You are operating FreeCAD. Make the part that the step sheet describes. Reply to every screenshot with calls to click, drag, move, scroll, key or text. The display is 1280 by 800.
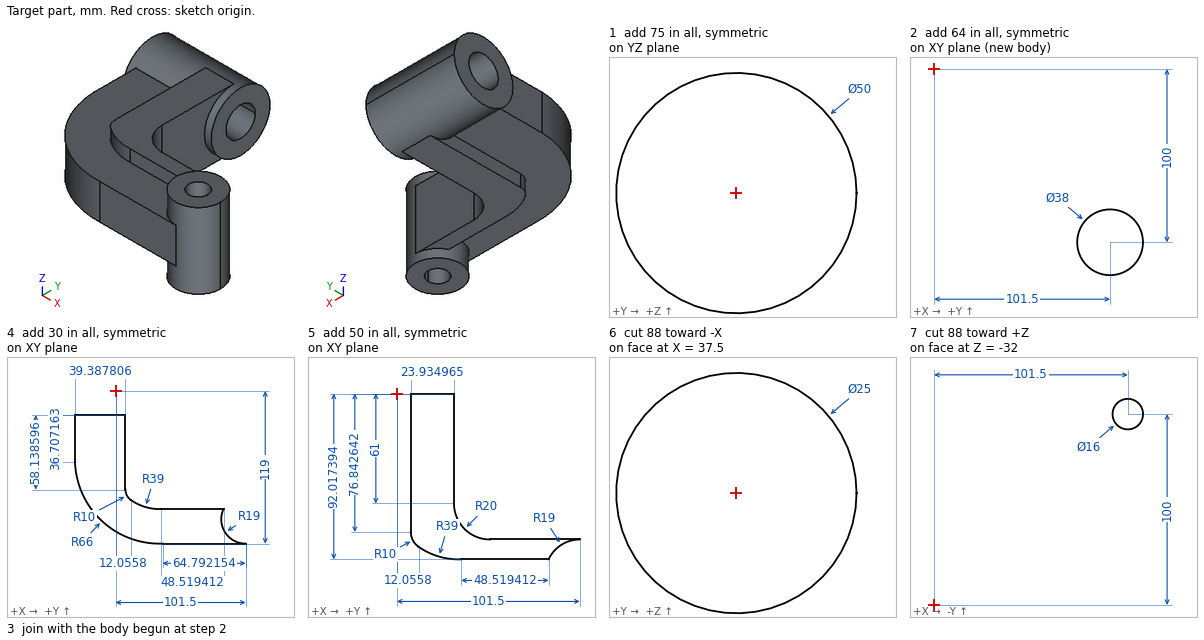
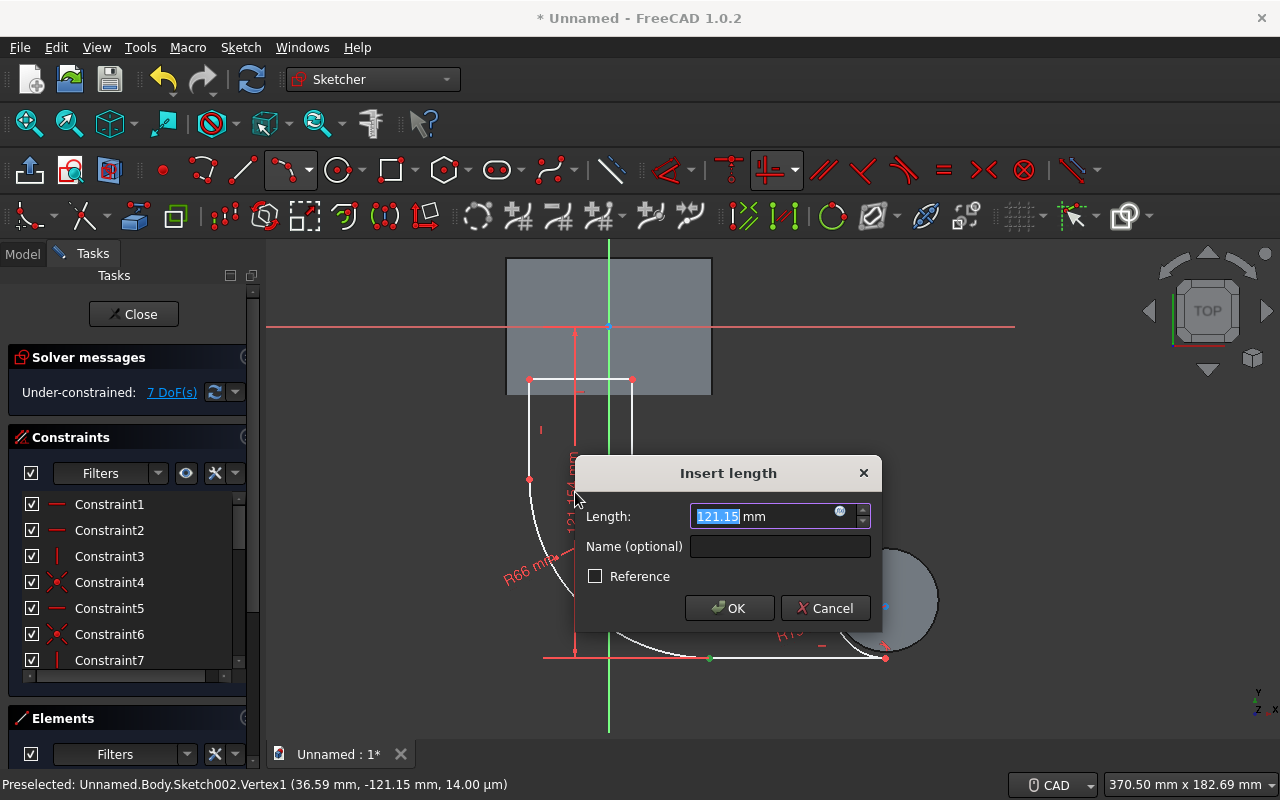
text(119)
key(Return)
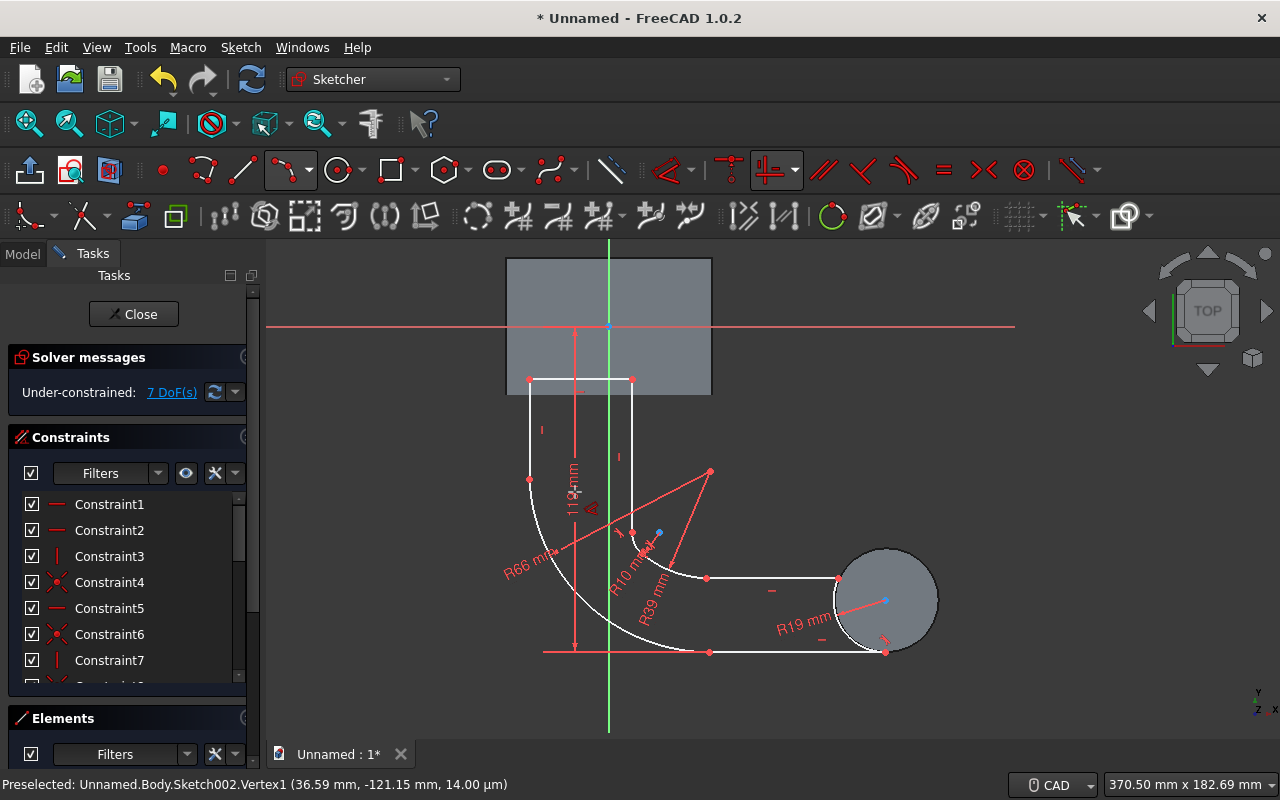
click(886, 652)
click(747, 686)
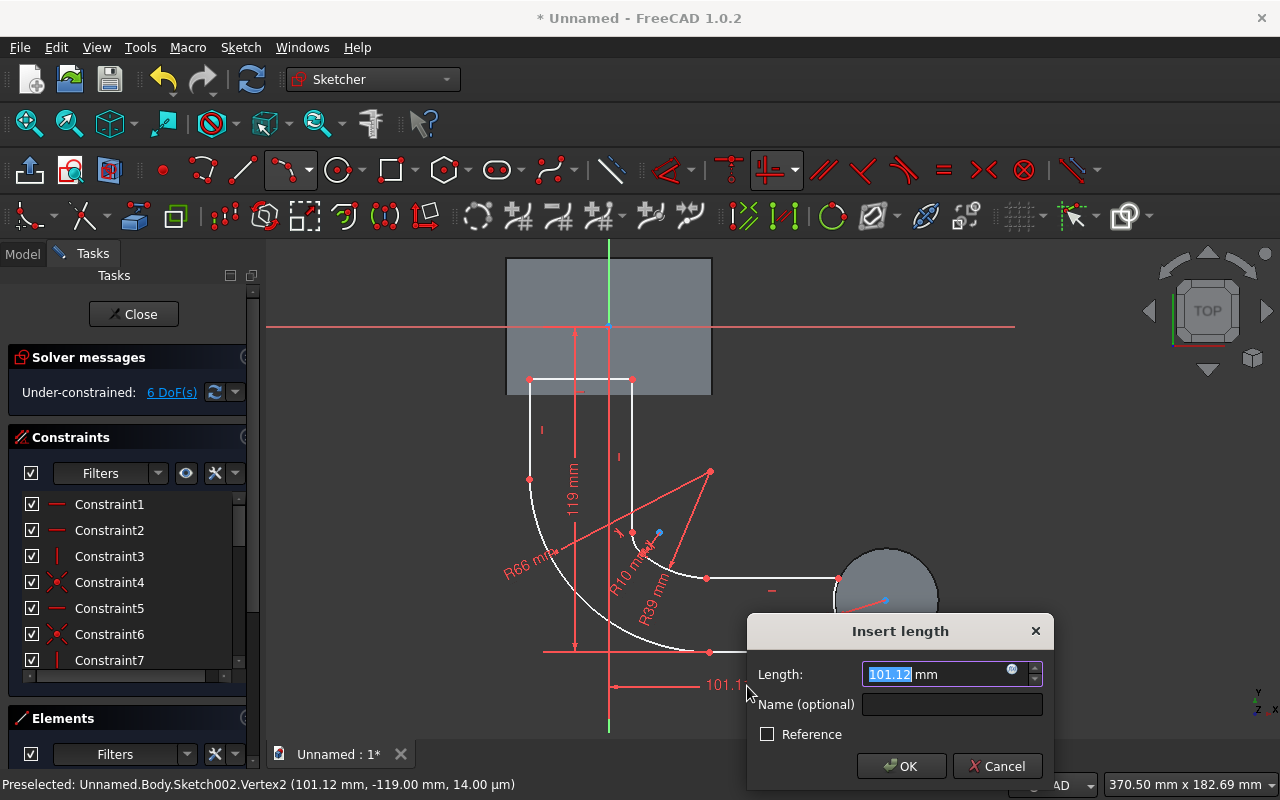
text(101.5)
key(Return)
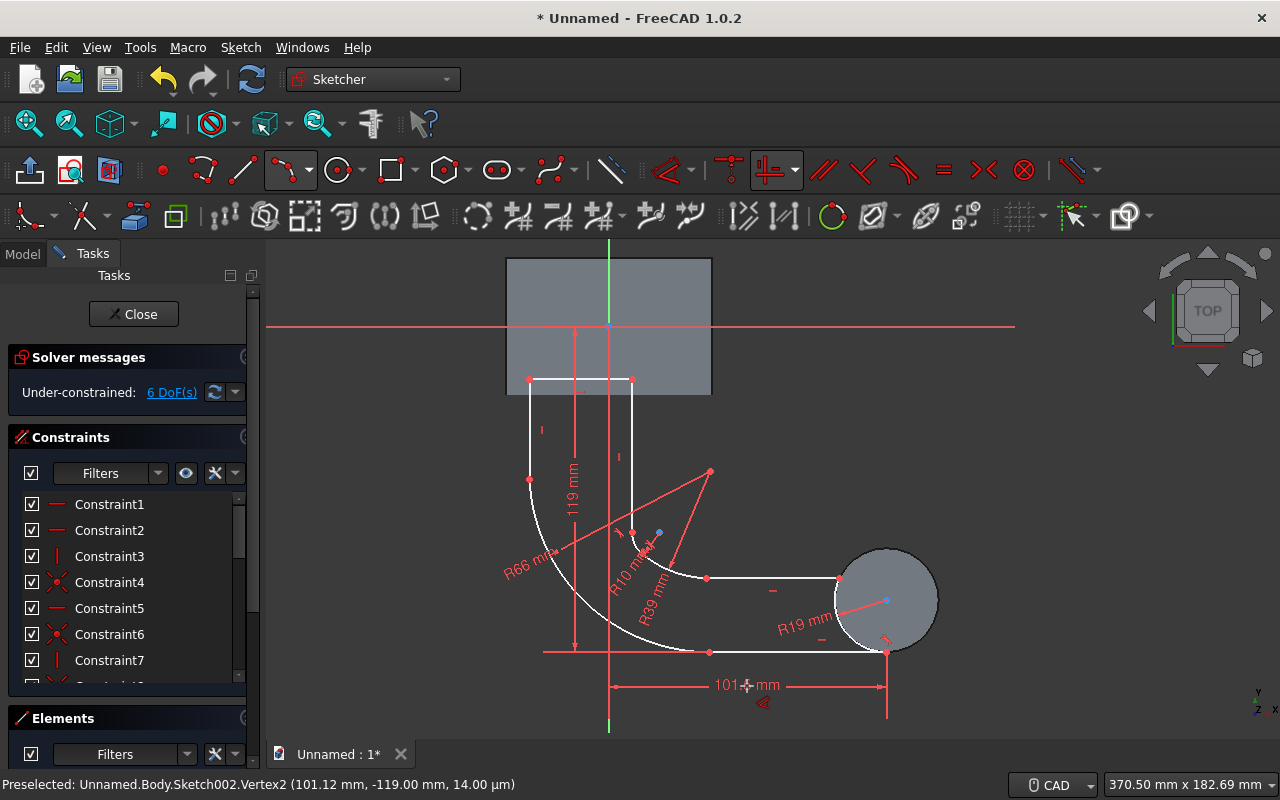
click(642, 554)
click(626, 293)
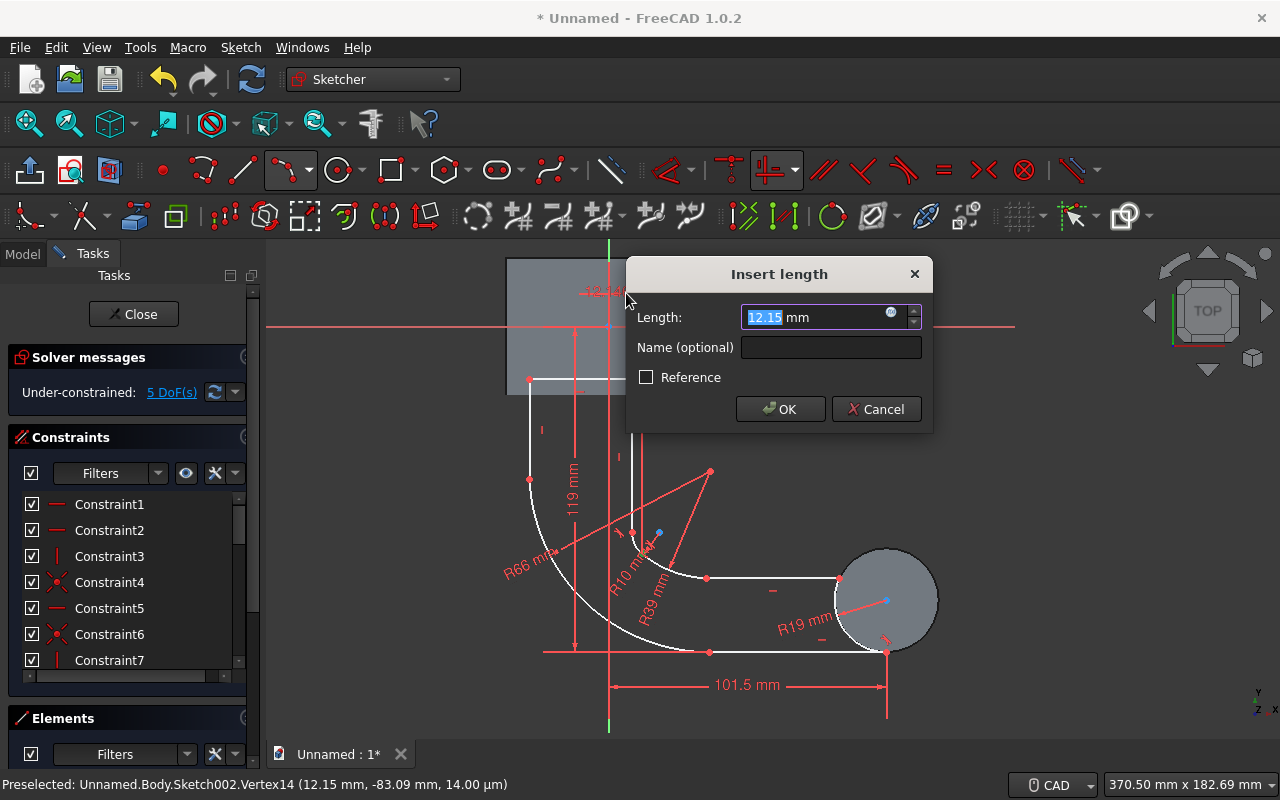
text(12.0558)
key(Return)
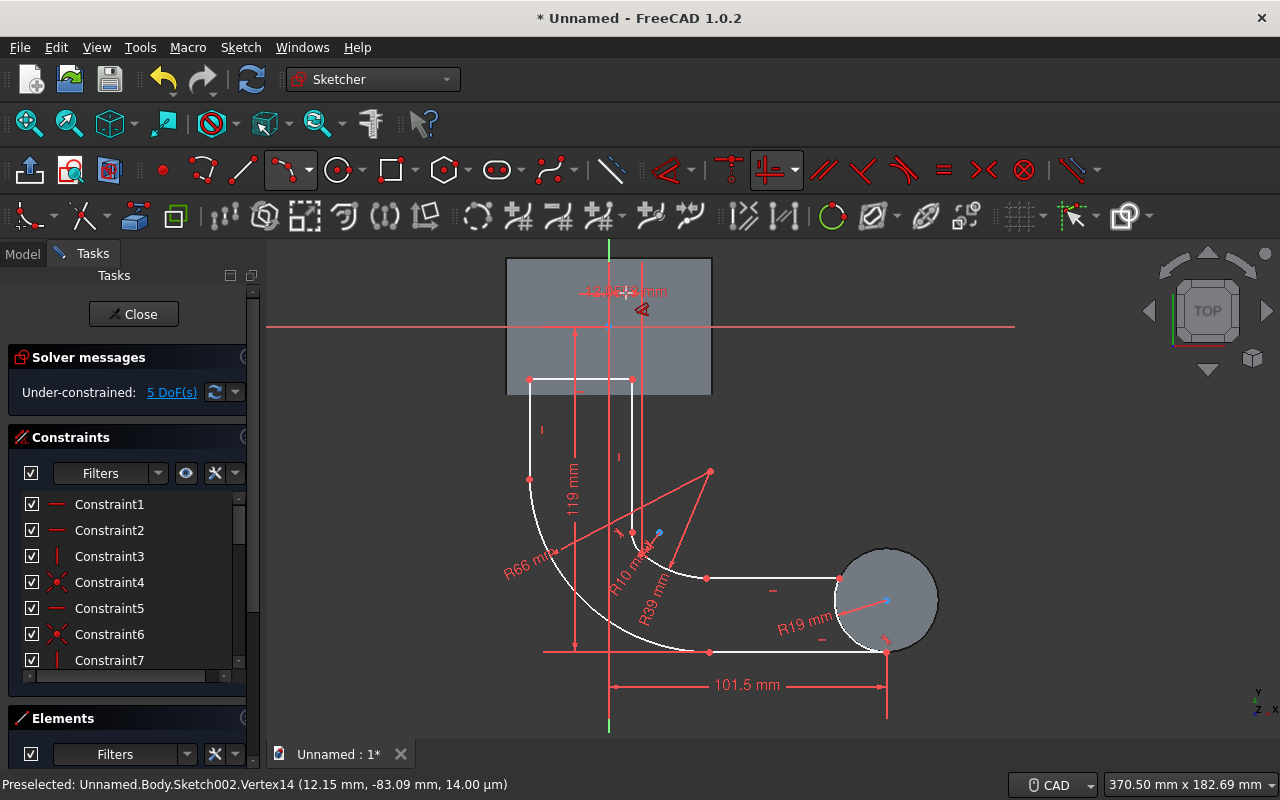
click(762, 652)
click(839, 686)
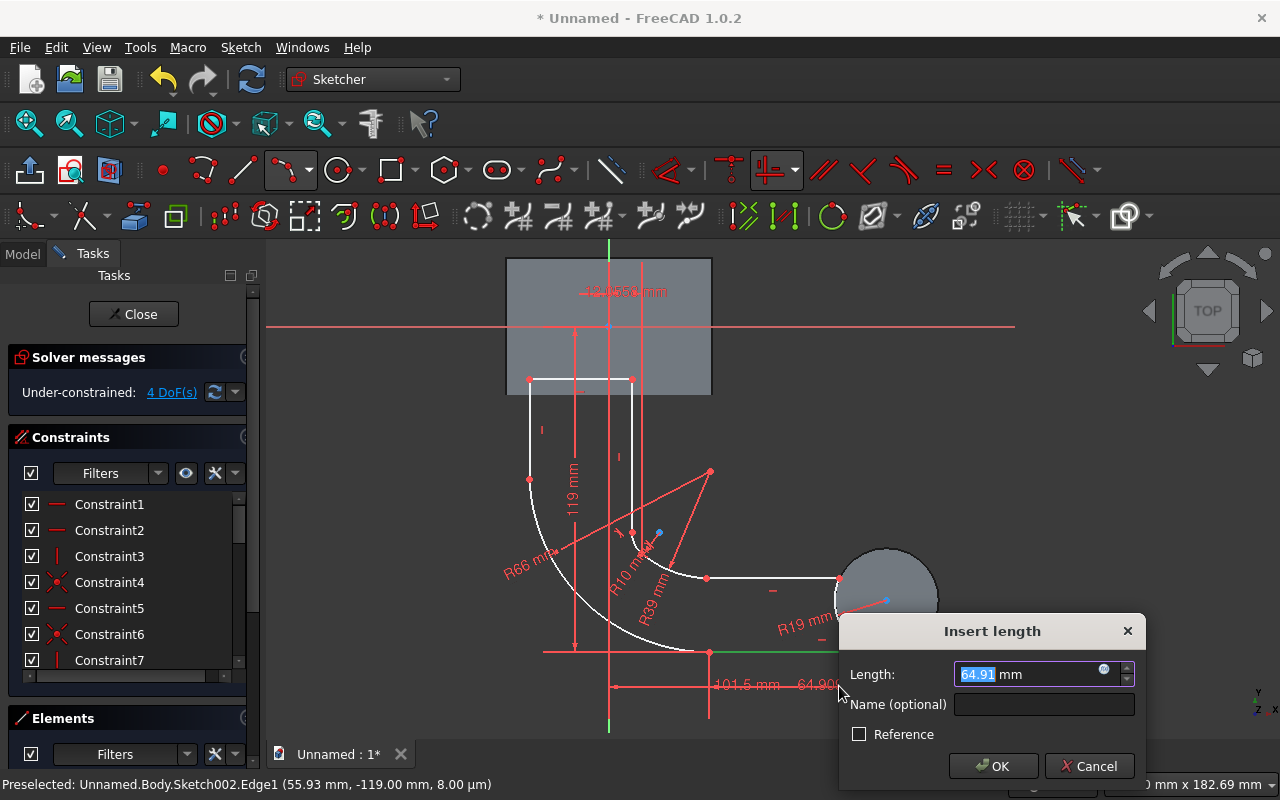
text(64.792154)
key(Return)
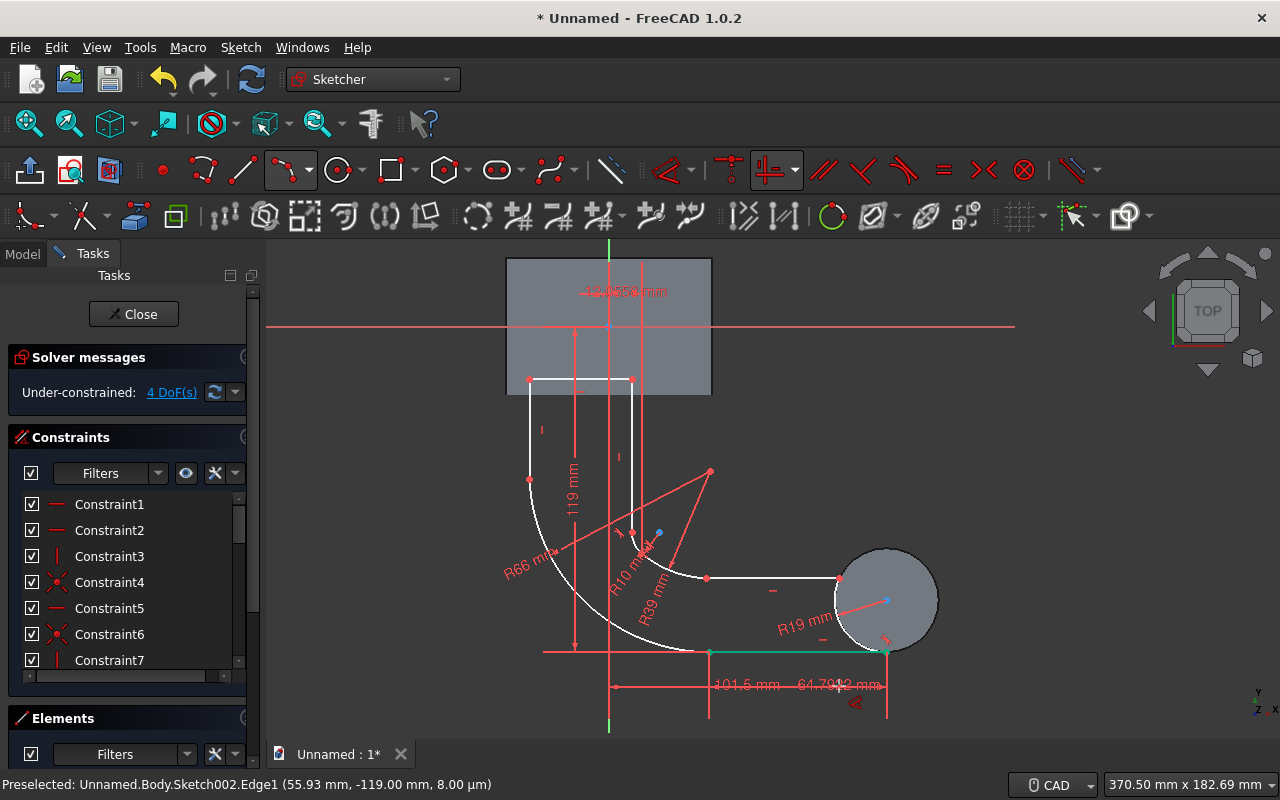
click(800, 578)
click(727, 612)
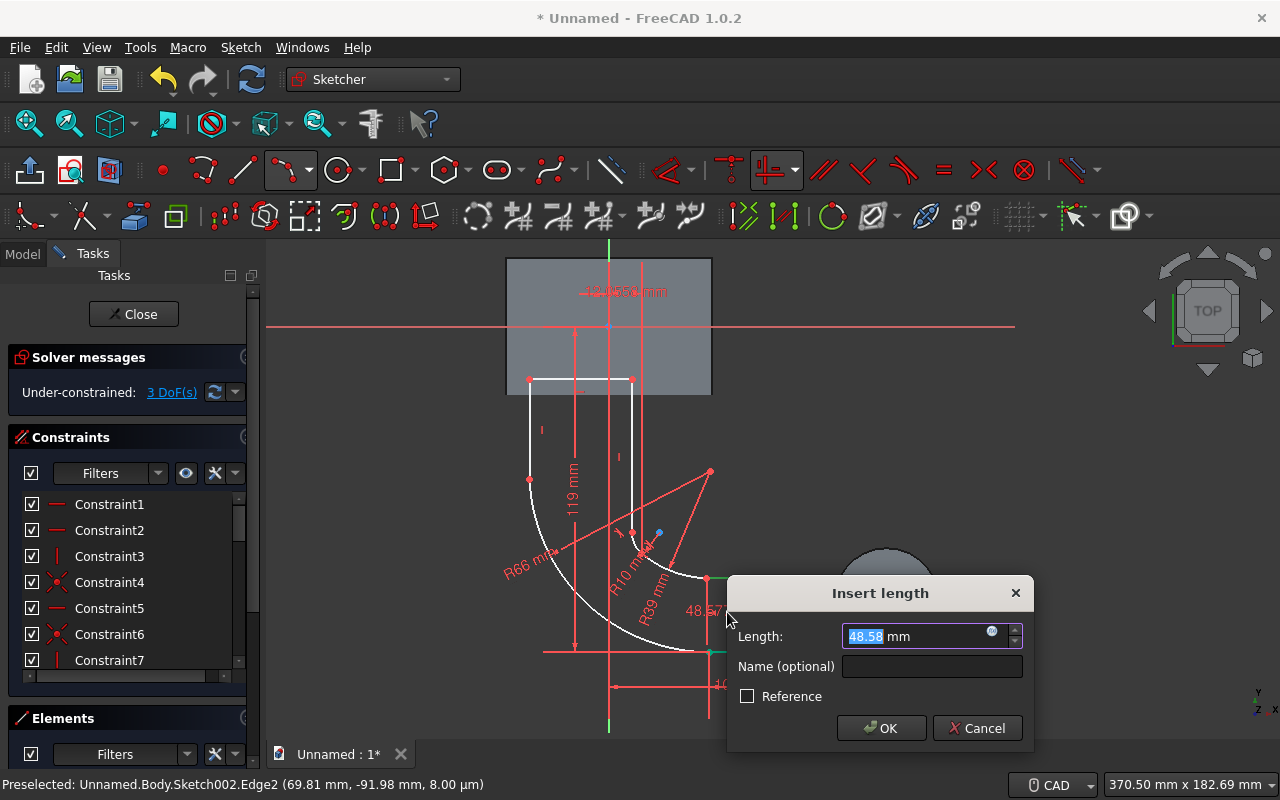
text(48.519412)
key(Return)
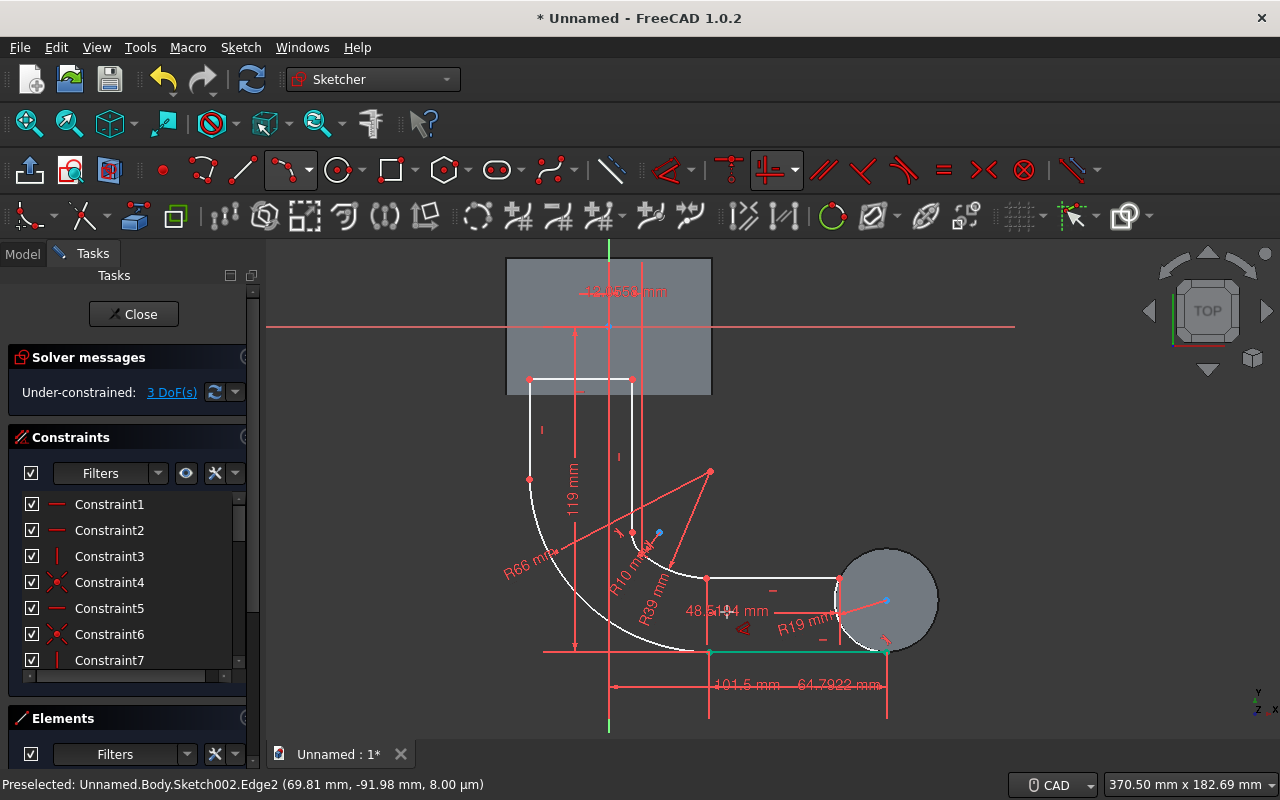
click(632, 487)
click(666, 456)